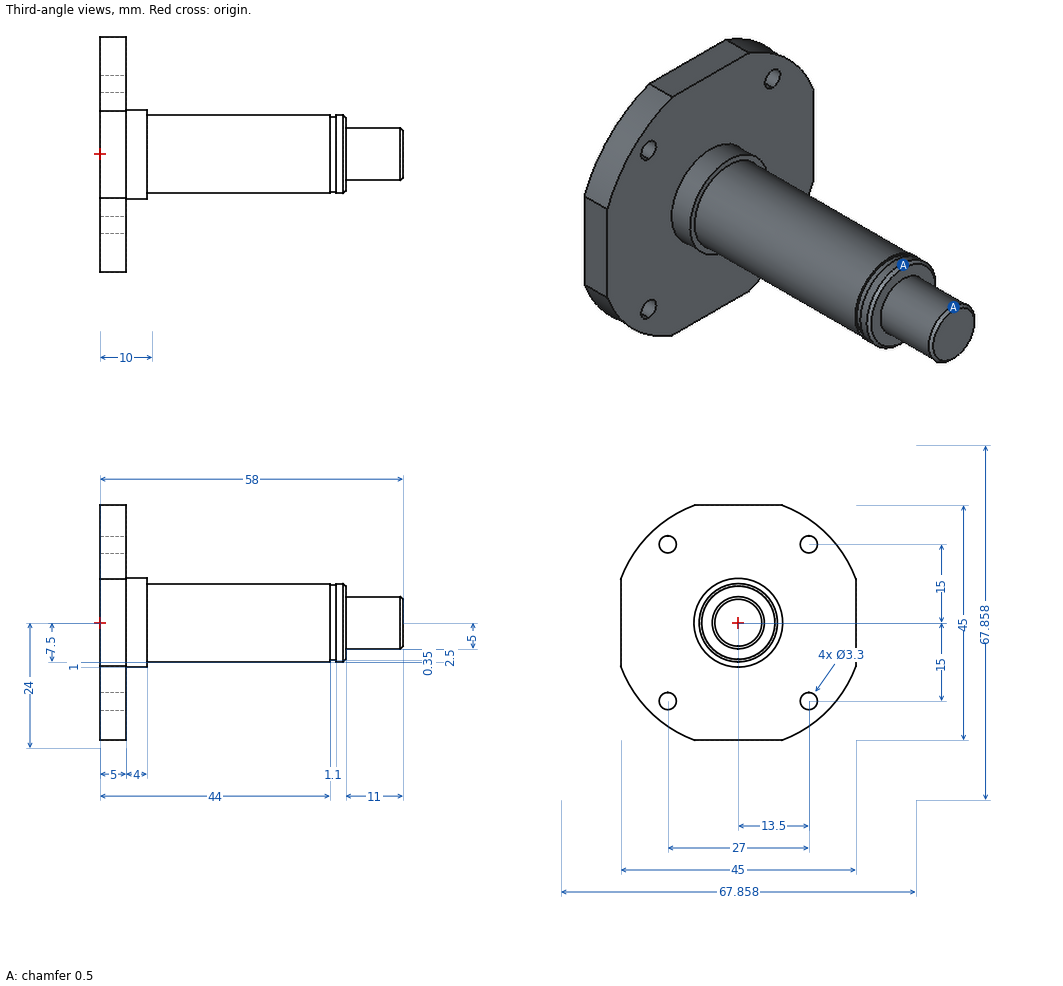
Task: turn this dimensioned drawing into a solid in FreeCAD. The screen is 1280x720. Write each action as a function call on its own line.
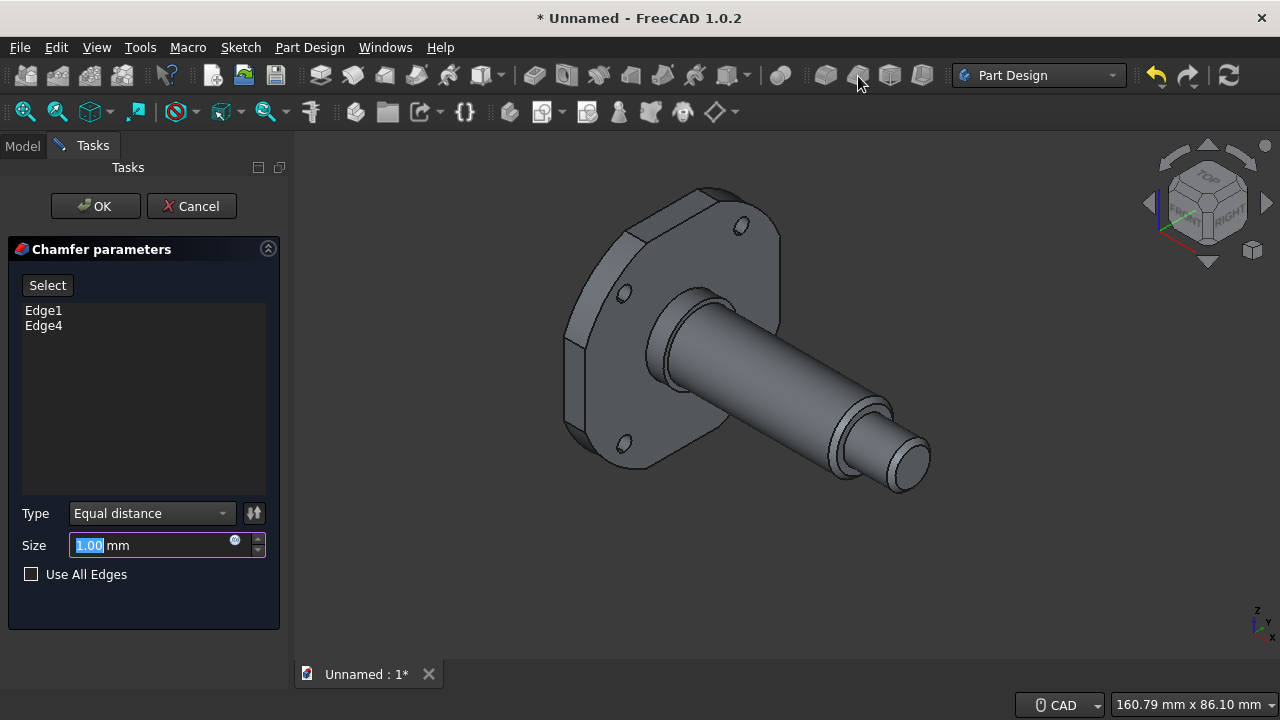
text(0.5)
key(Tab)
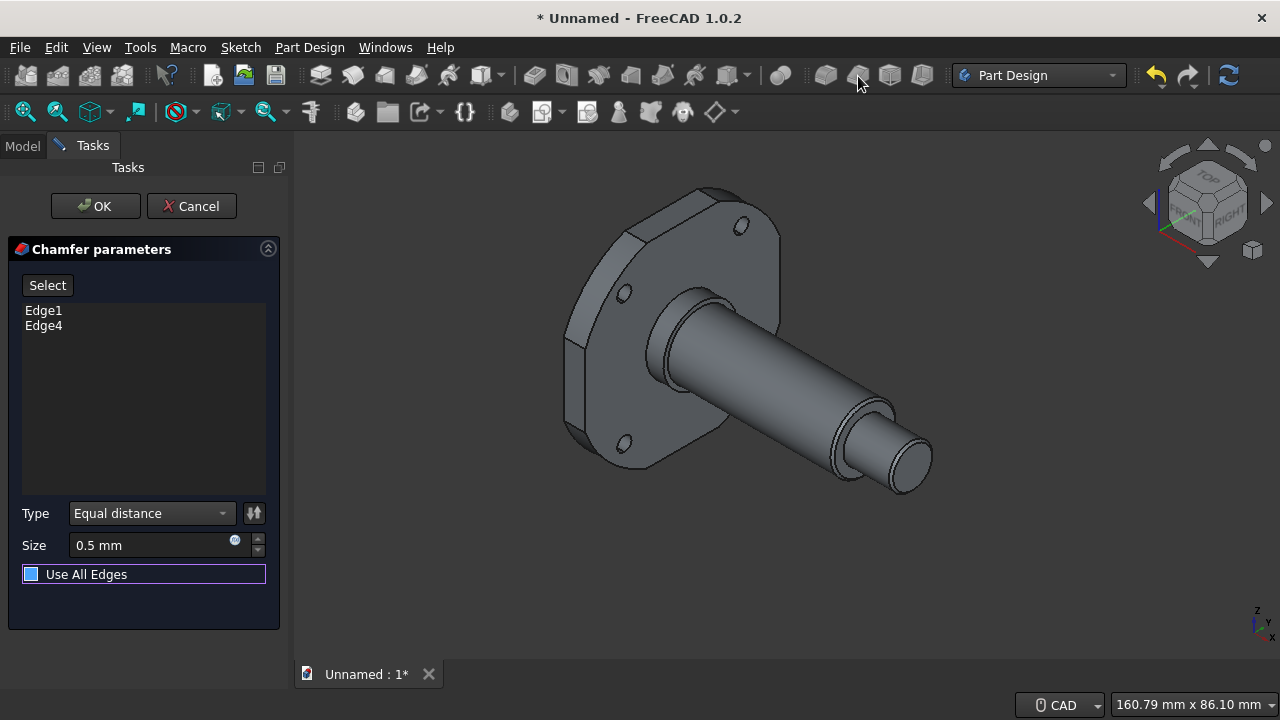
click(96, 206)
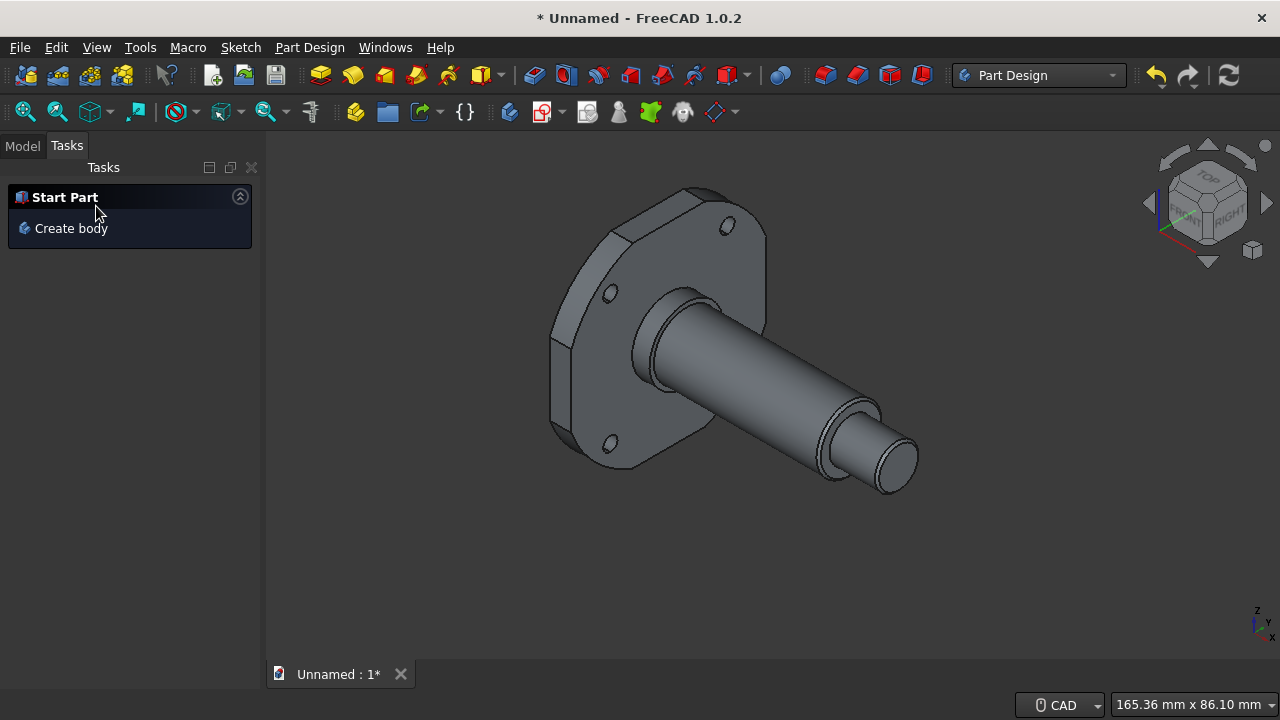
click(542, 112)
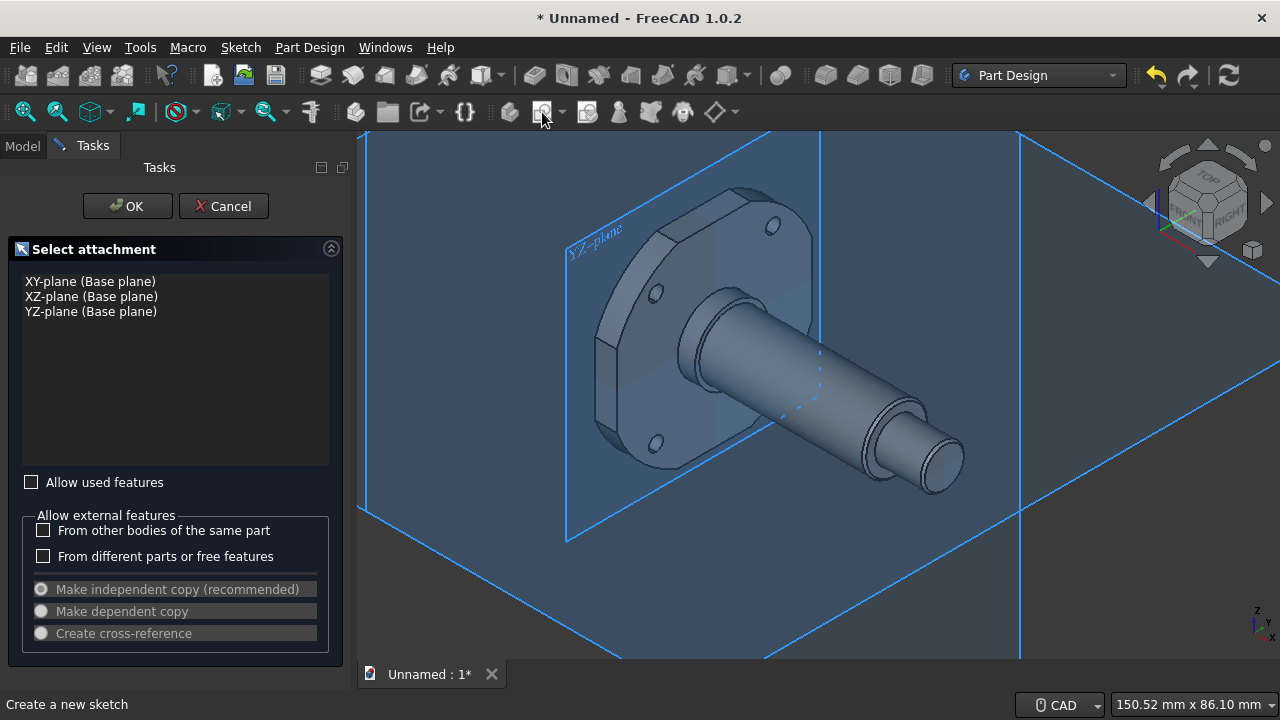
click(82, 296)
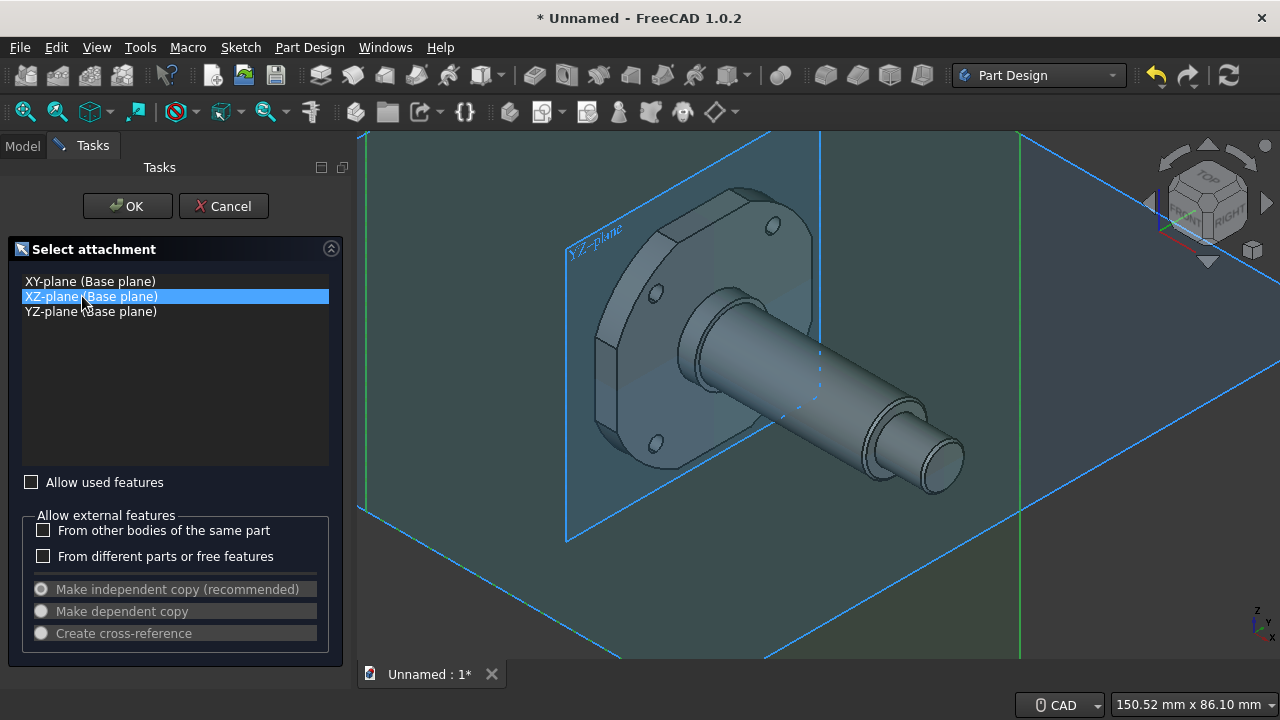
click(128, 206)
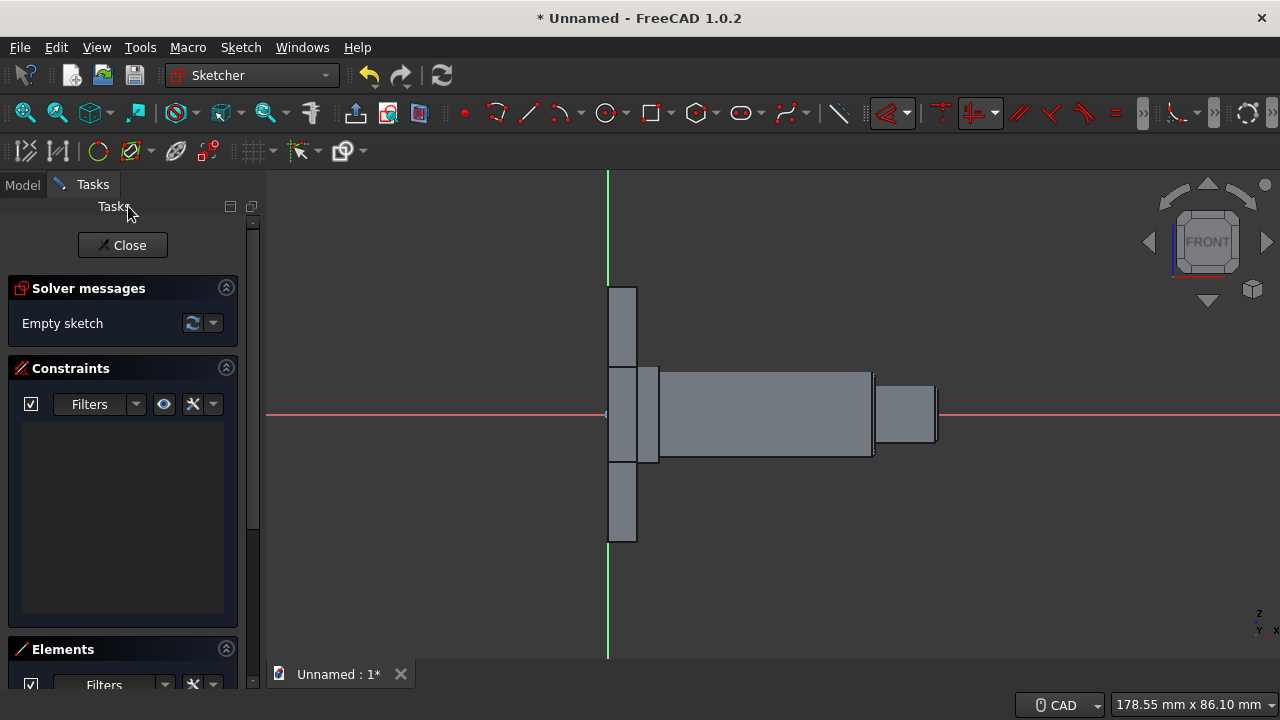
click(420, 114)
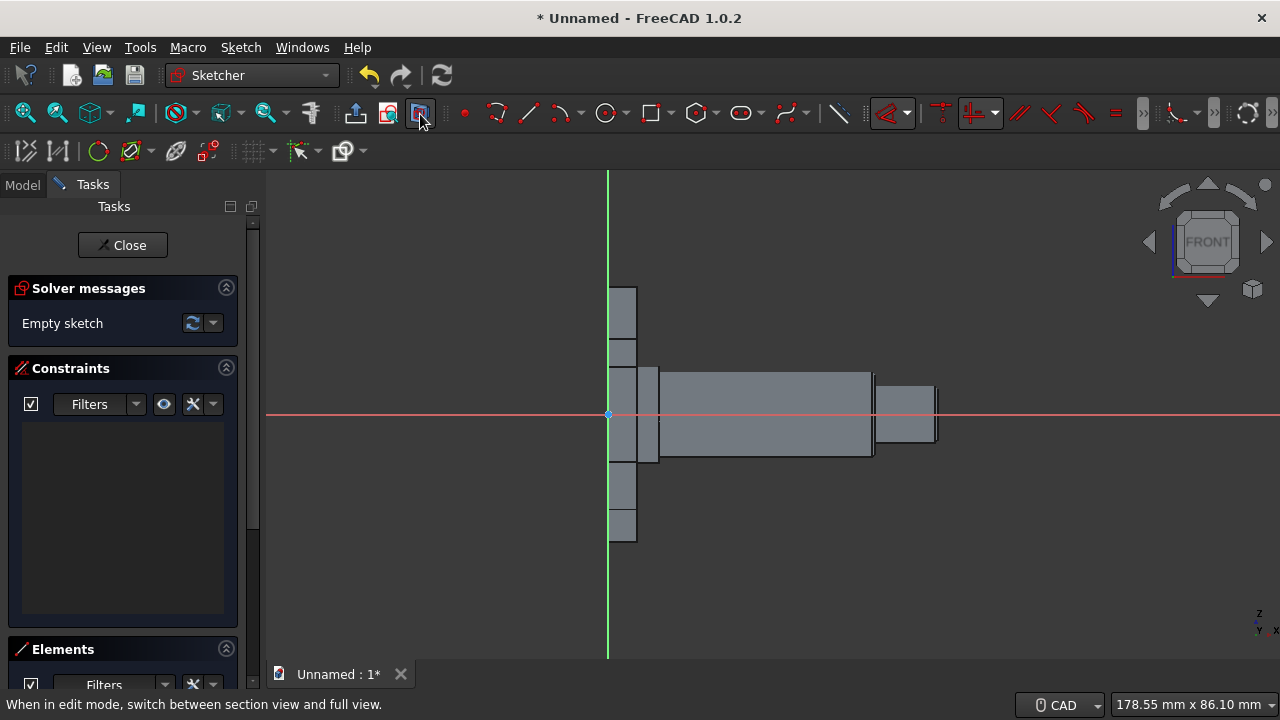
scroll(870, 458, up, 15)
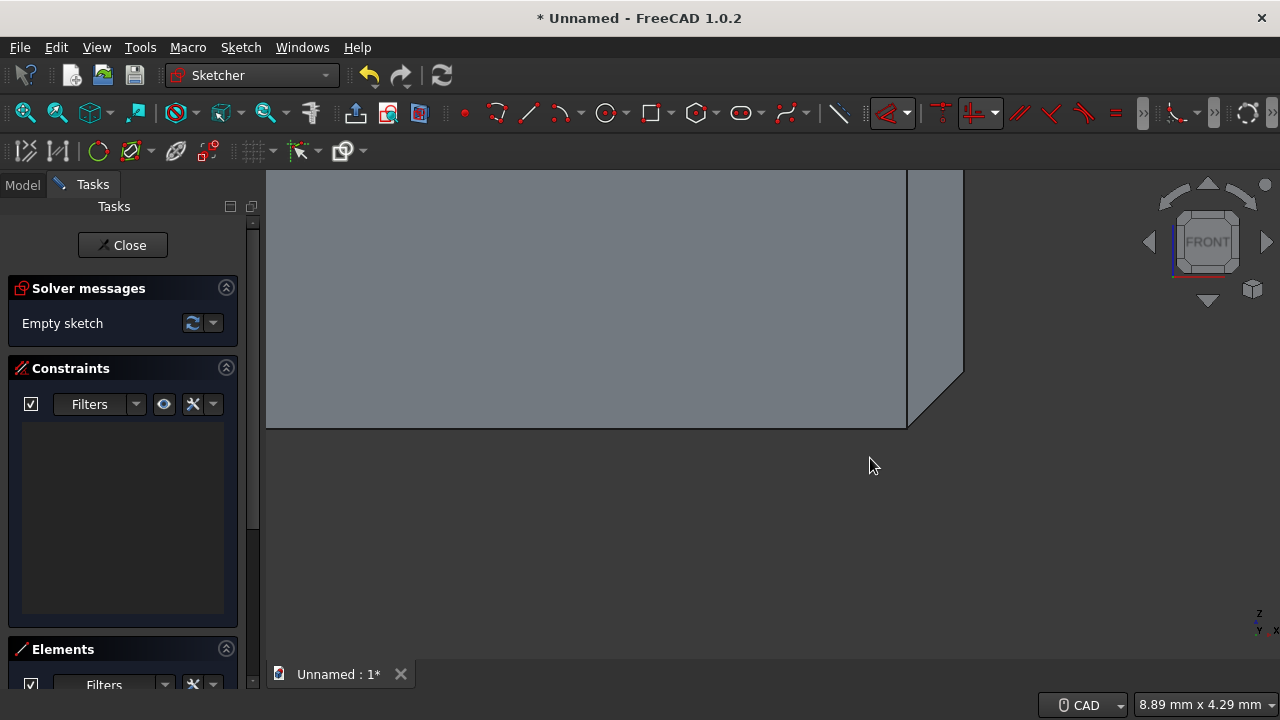
scroll(679, 407, up, 8)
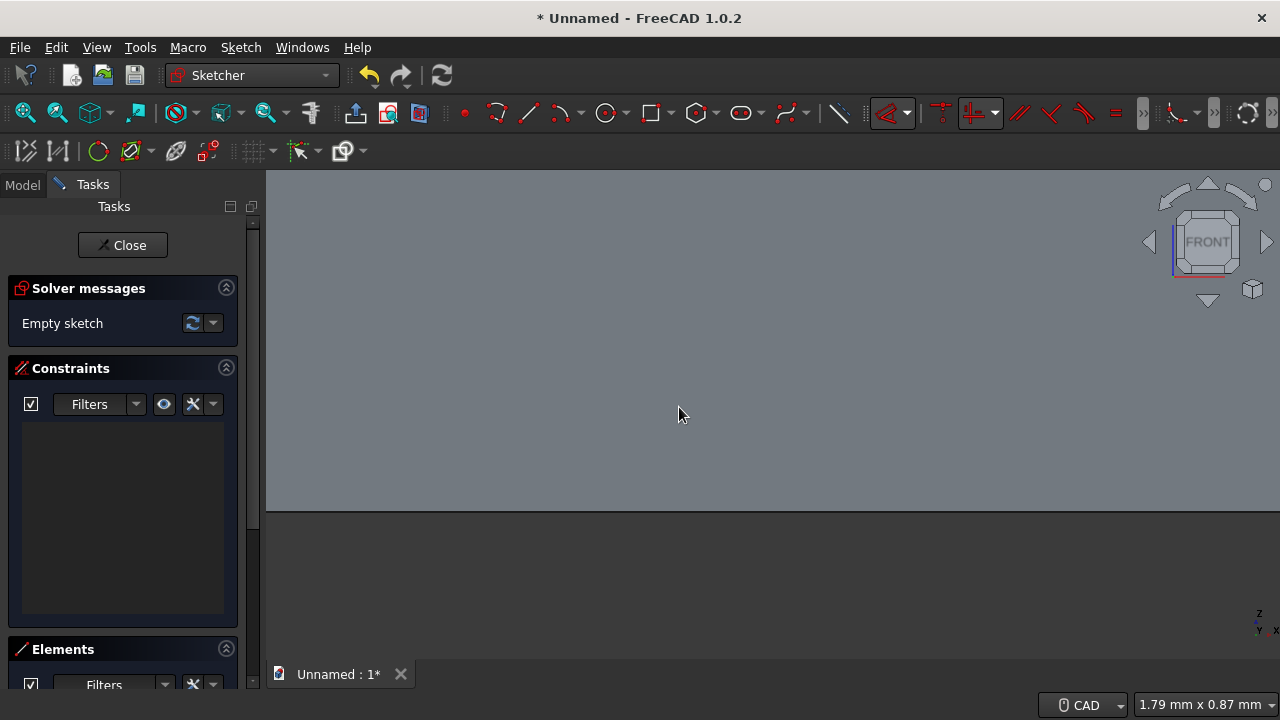
click(652, 114)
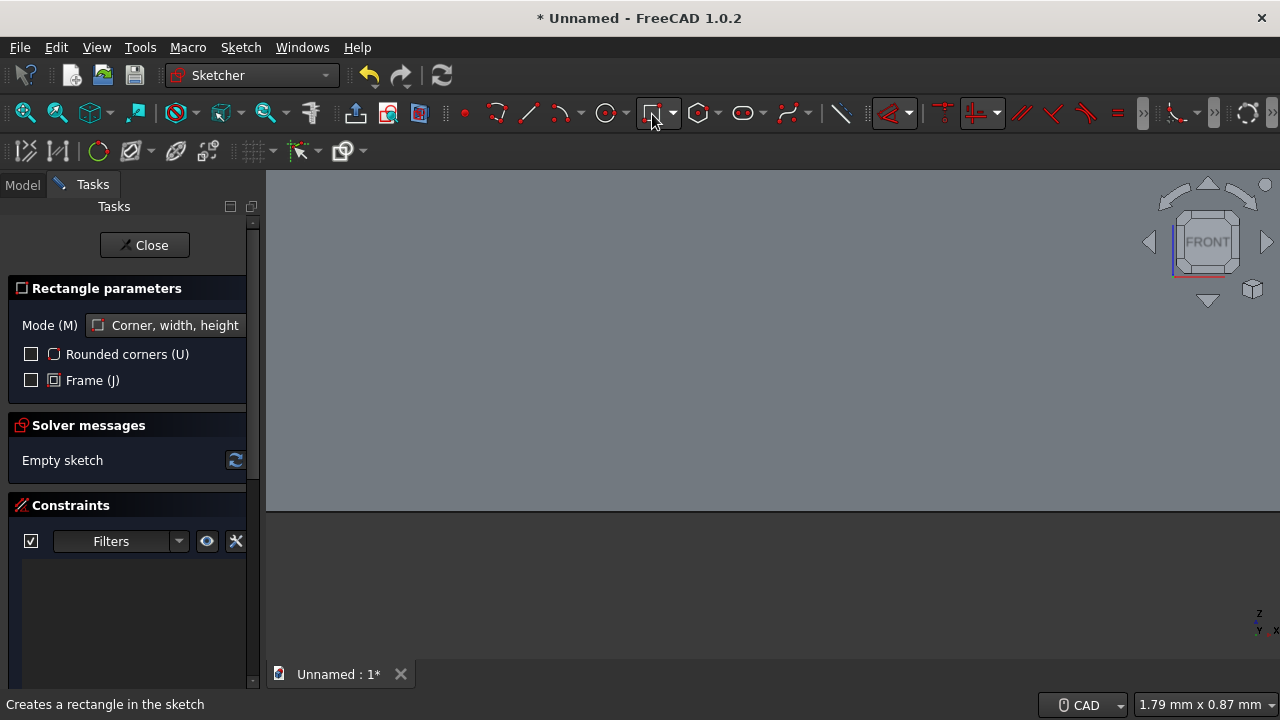
click(392, 314)
click(1013, 512)
key(Escape)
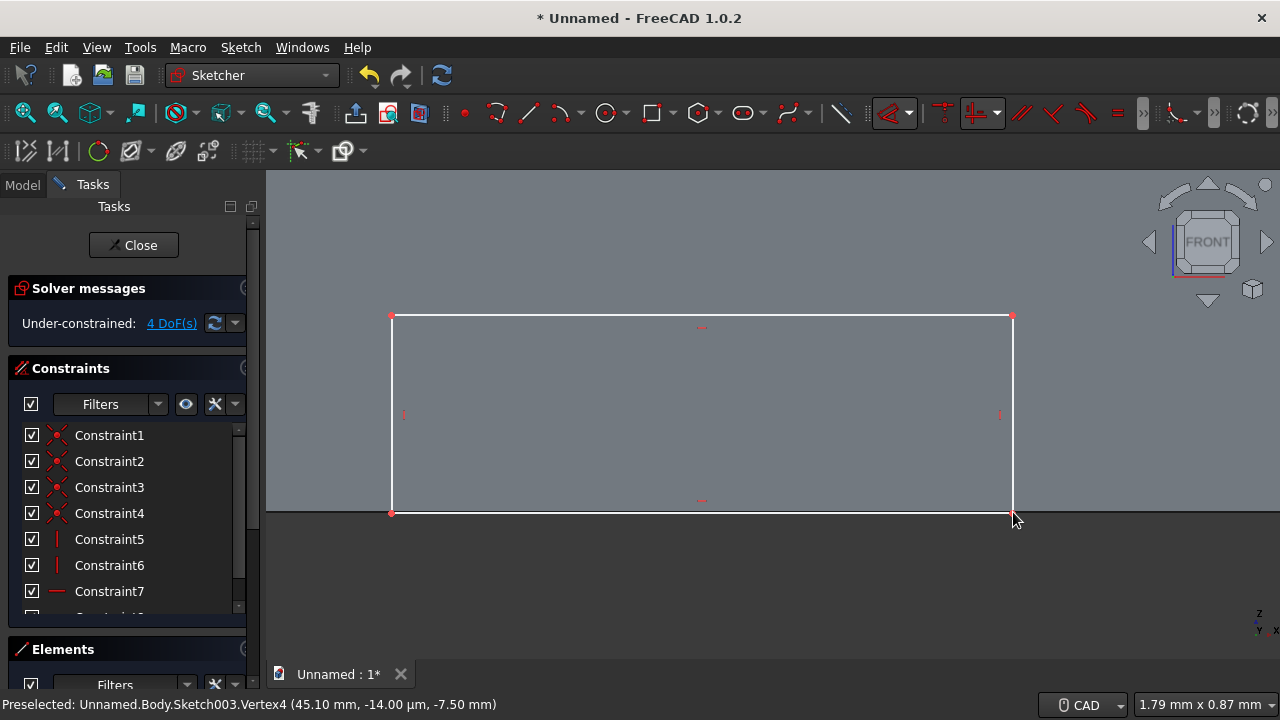
click(578, 513)